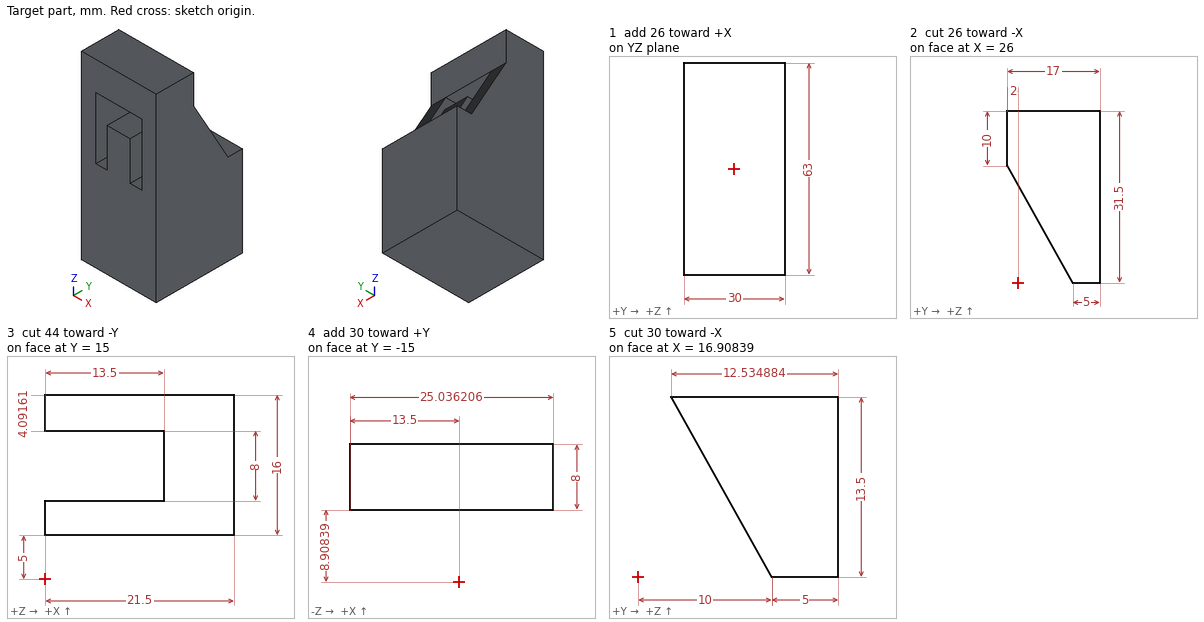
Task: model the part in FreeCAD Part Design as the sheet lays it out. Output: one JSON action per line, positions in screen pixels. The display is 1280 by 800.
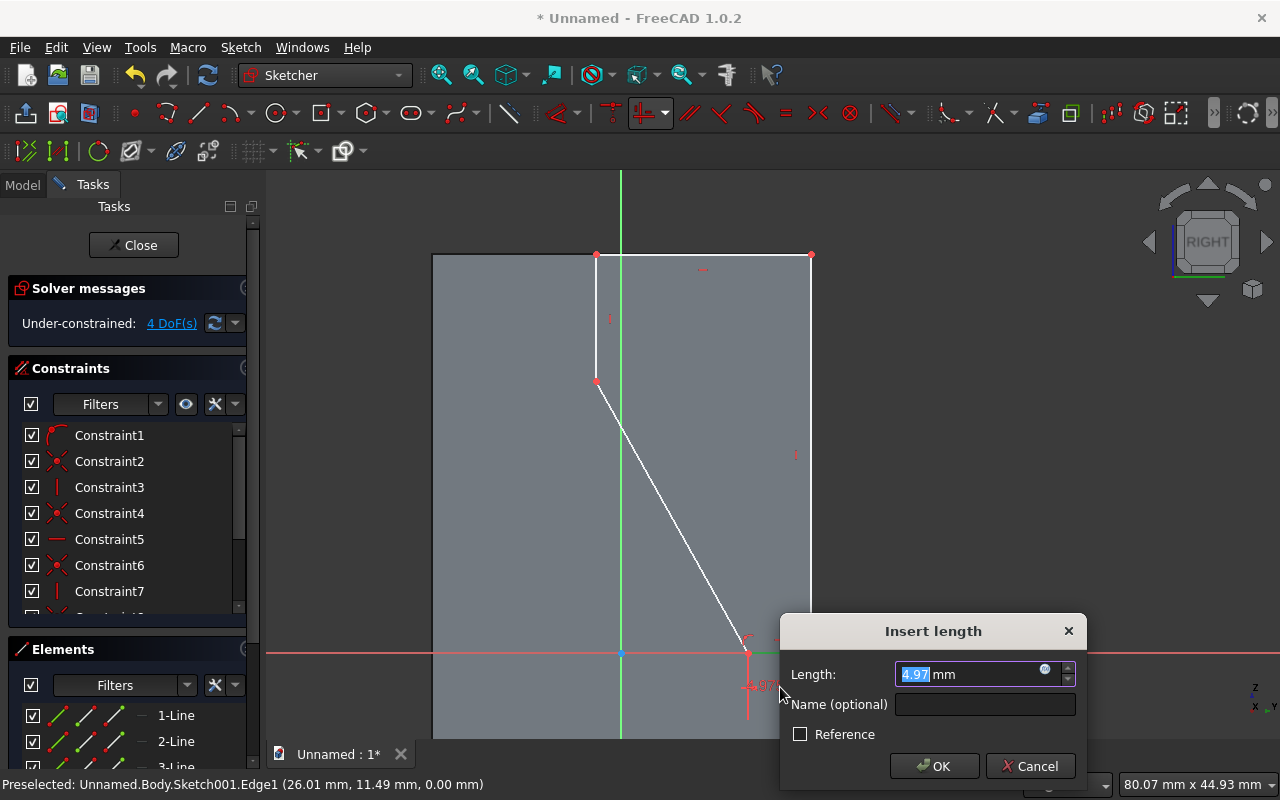
{"action": "type", "text": "5"}
{"action": "key", "text": "Return"}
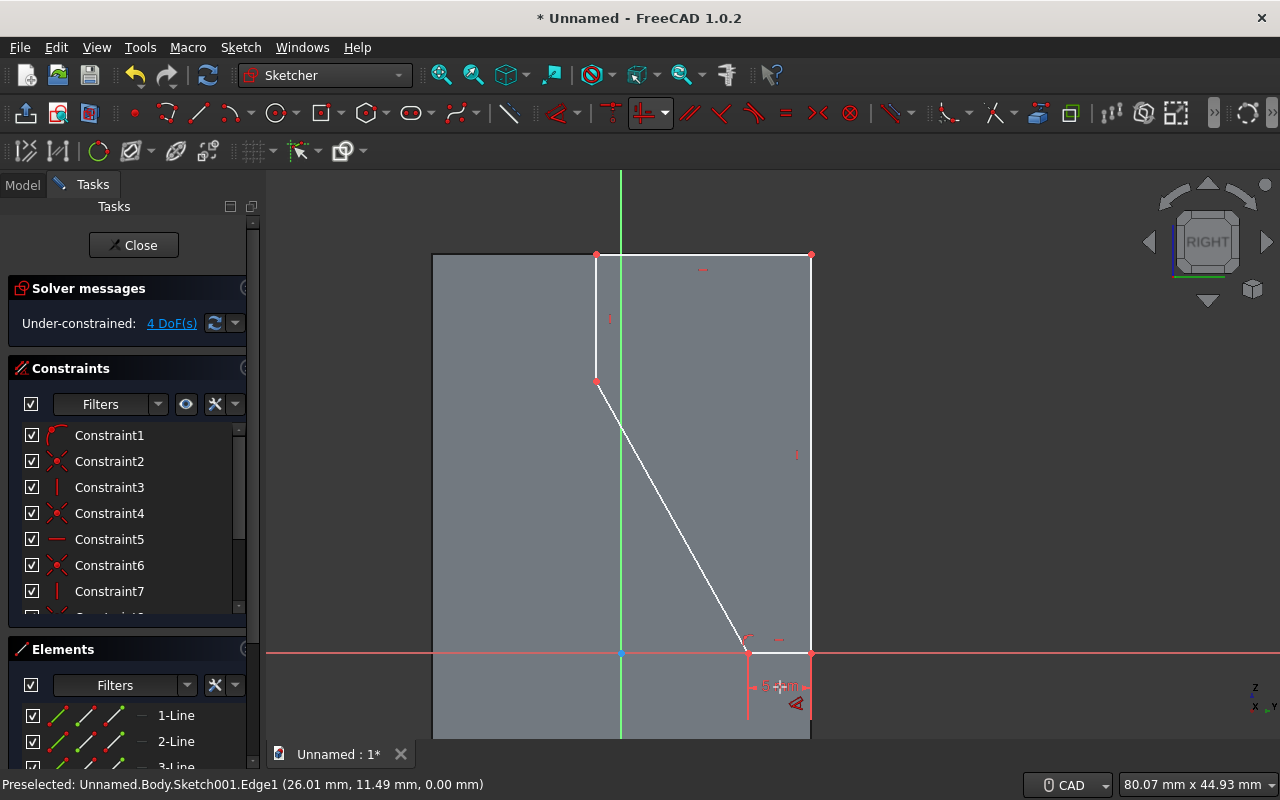
{"action": "left_click", "coordinate": [747, 255]}
{"action": "left_click", "coordinate": [704, 221]}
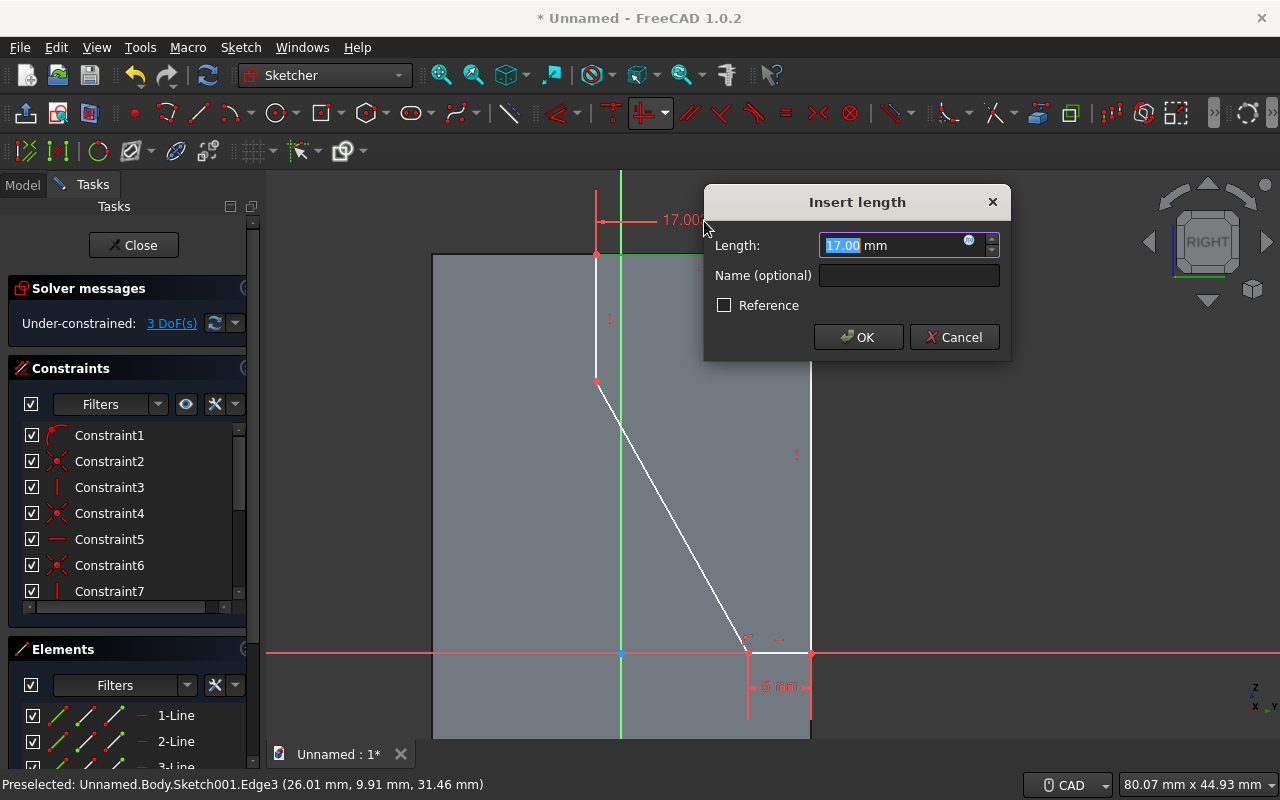
{"action": "type", "text": "17"}
{"action": "key", "text": "Return"}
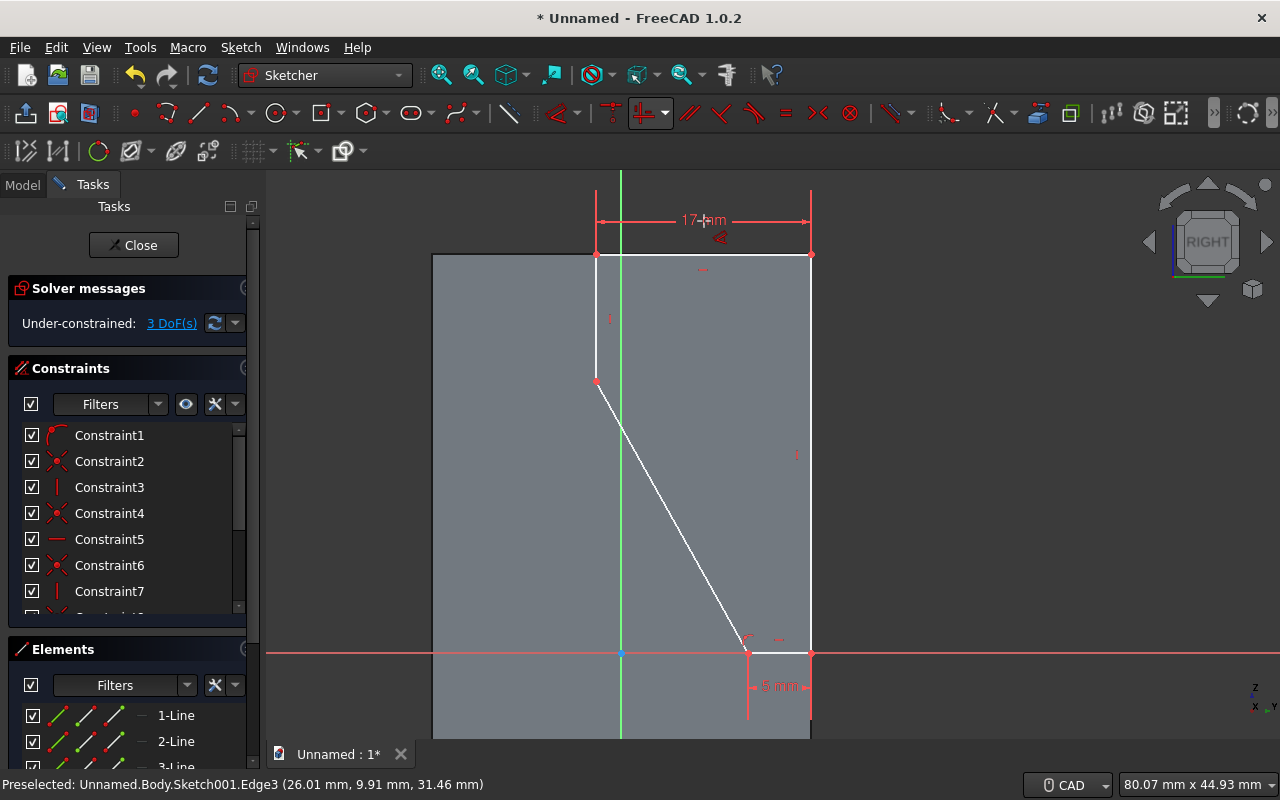
{"action": "left_click", "coordinate": [596, 293]}
{"action": "left_click", "coordinate": [562, 319]}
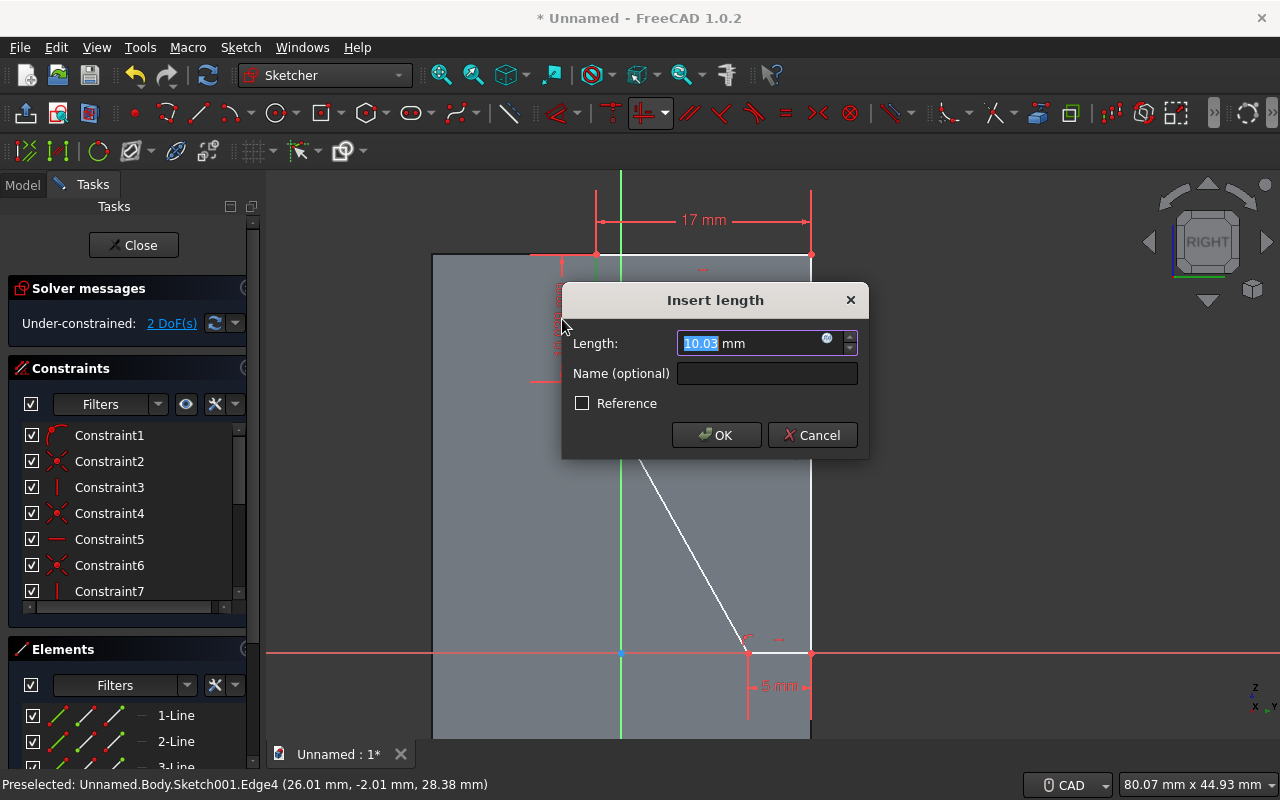
{"action": "type", "text": "10"}
{"action": "key", "text": "Return"}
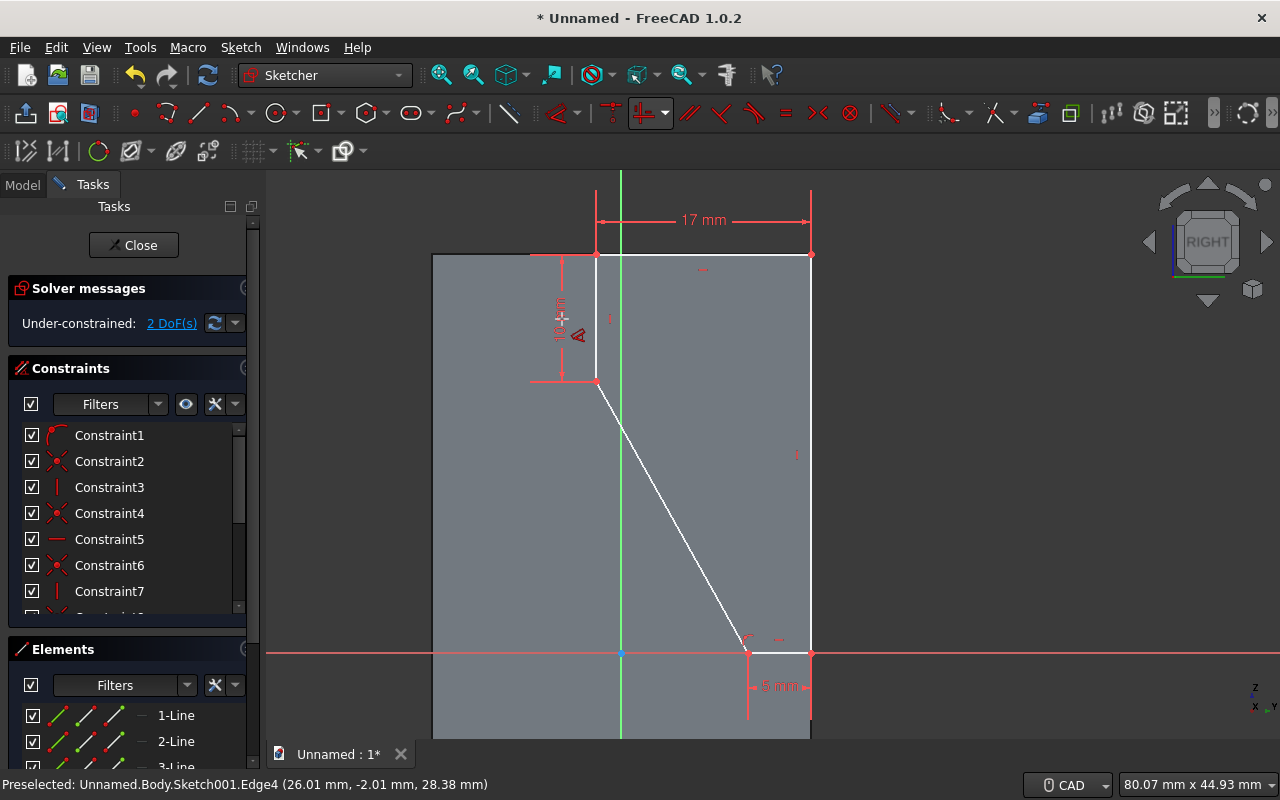
{"action": "scroll", "coordinate": [596, 255], "scroll_direction": "up", "scroll_amount": 3}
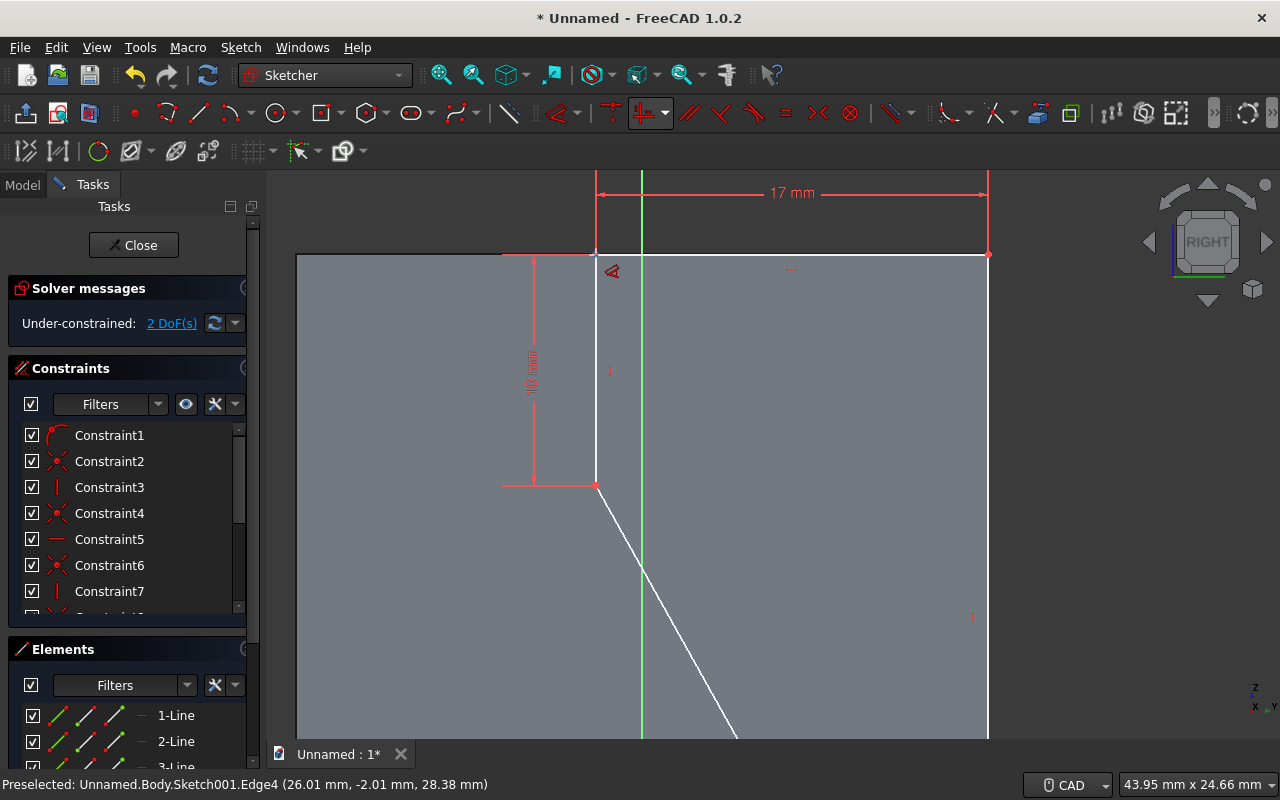
{"action": "left_click", "coordinate": [596, 255]}
{"action": "left_click", "coordinate": [619, 221]}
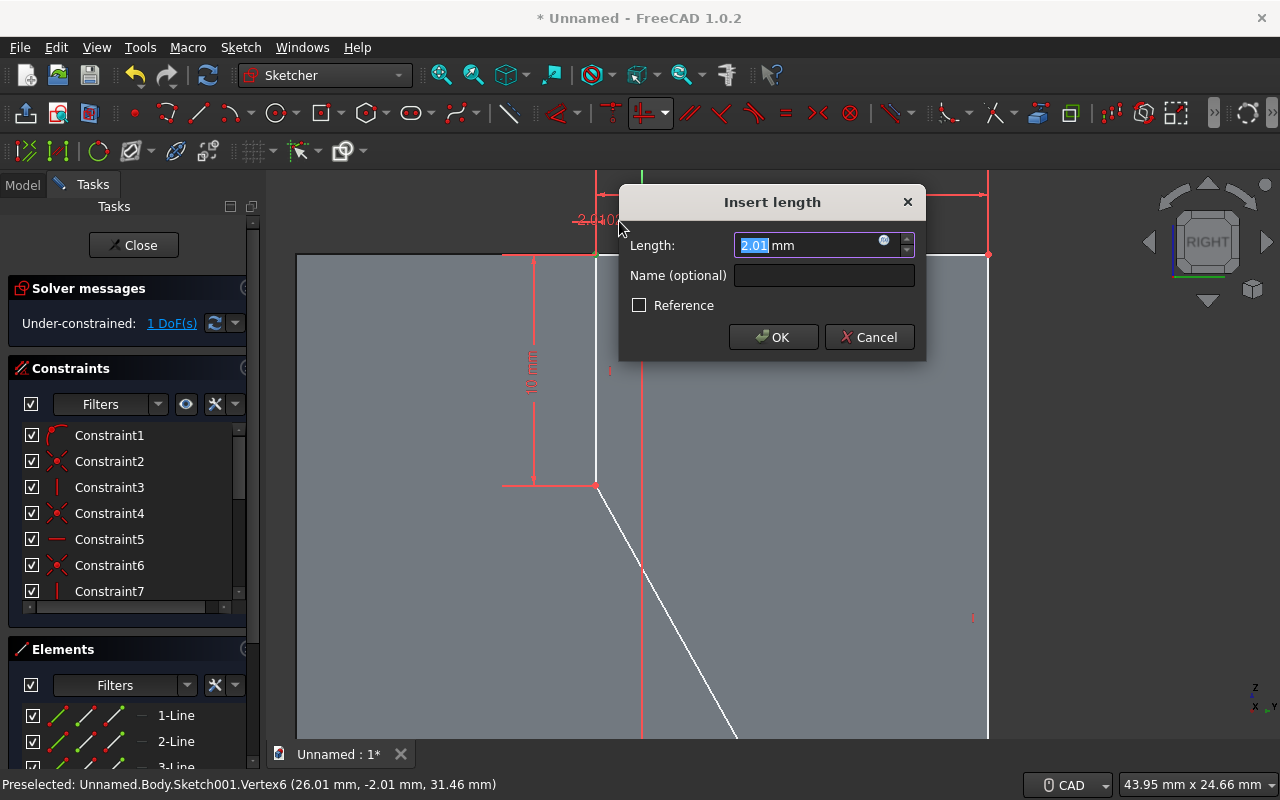
{"action": "type", "text": "2"}
{"action": "key", "text": "Return"}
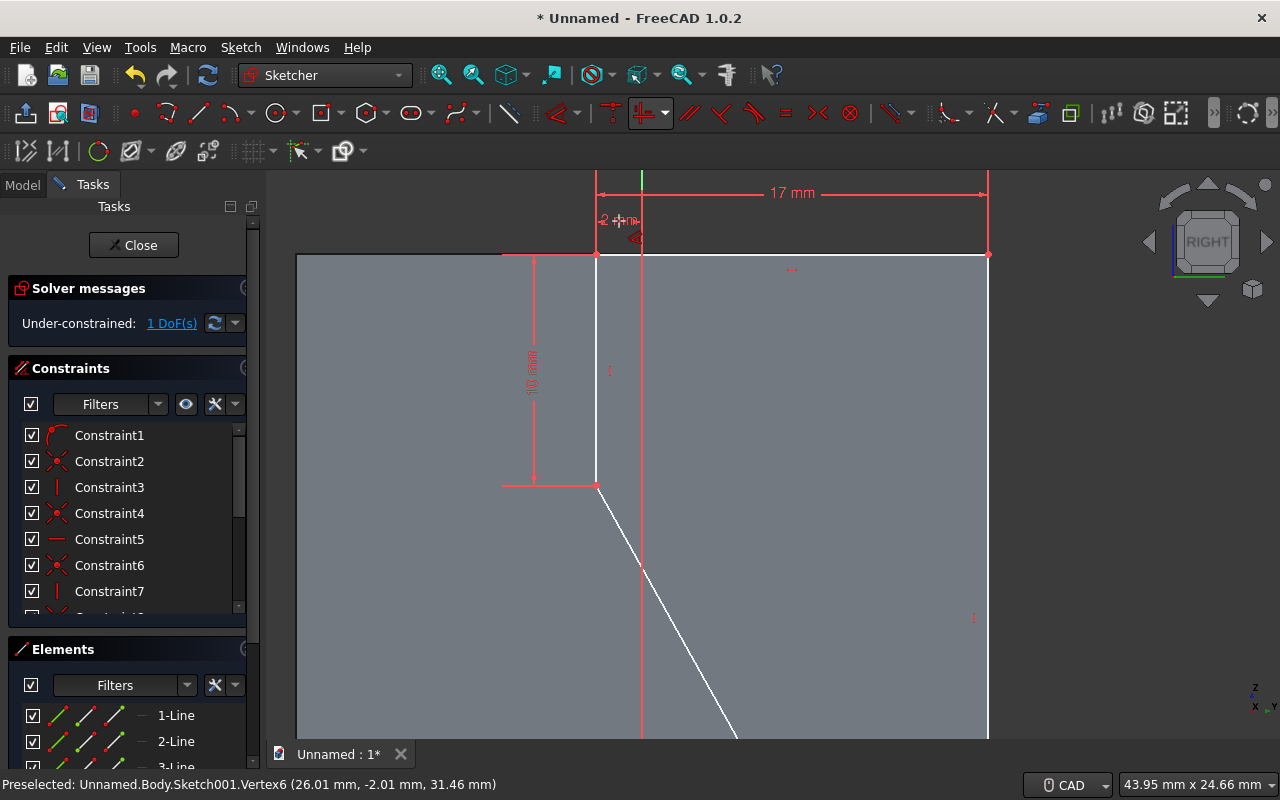
{"action": "left_click", "coordinate": [988, 473]}
{"action": "left_click", "coordinate": [1022, 483]}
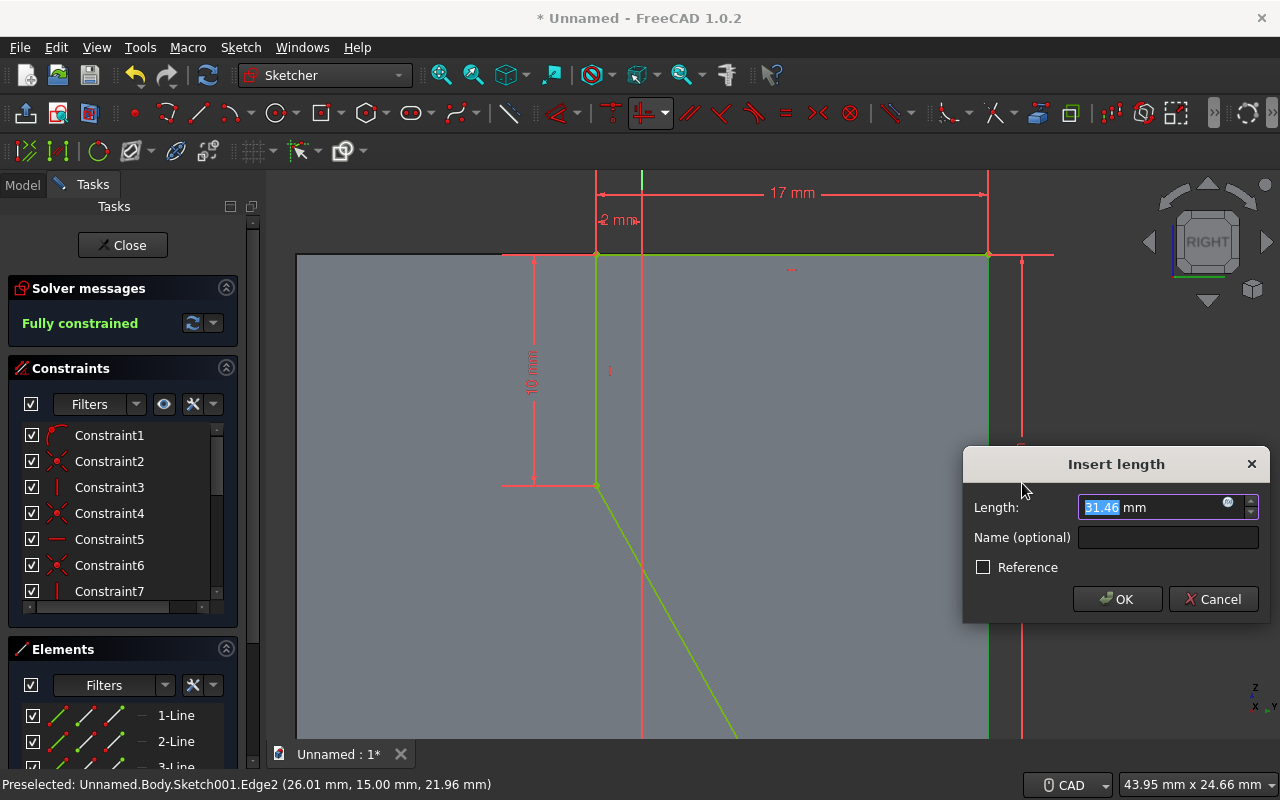
{"action": "type", "text": "31.5"}
{"action": "key", "text": "Return"}
{"action": "key", "text": "Escape"}